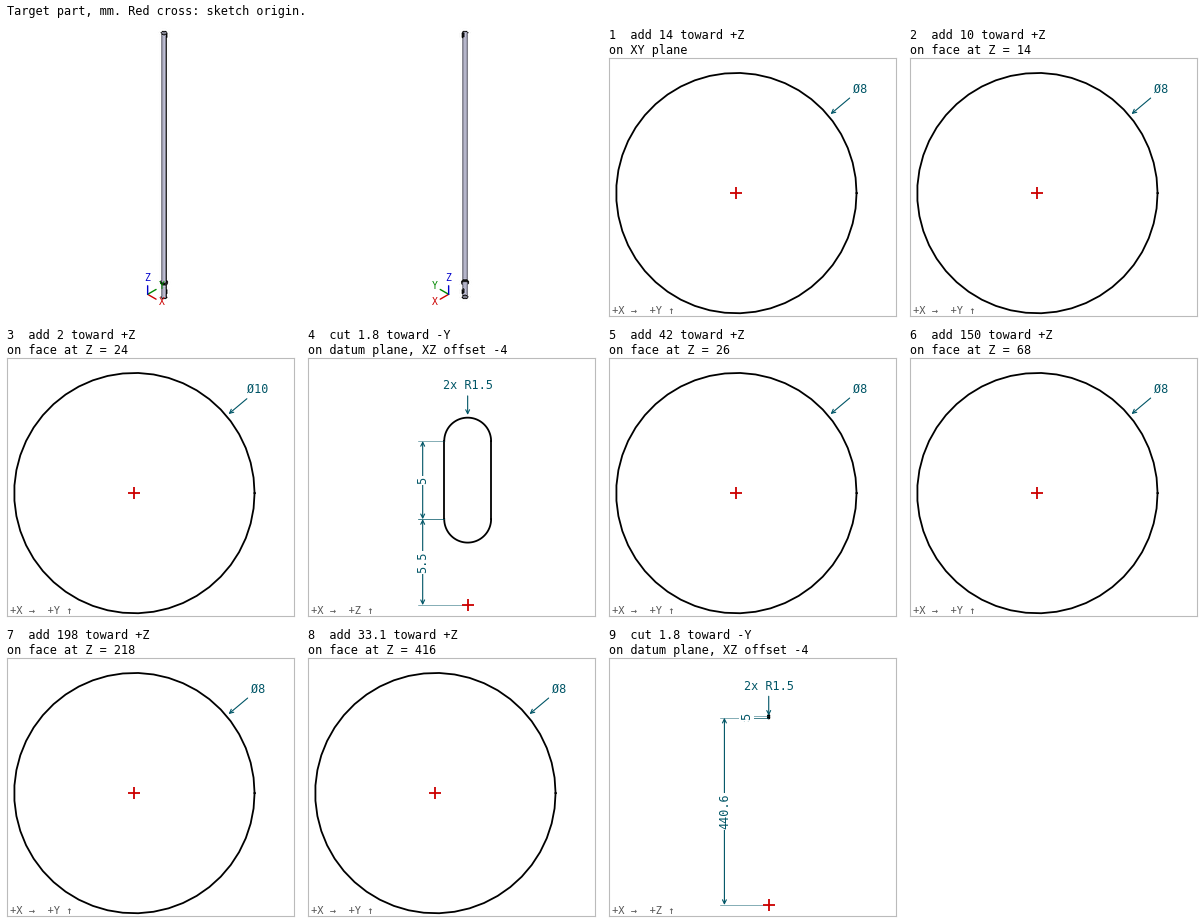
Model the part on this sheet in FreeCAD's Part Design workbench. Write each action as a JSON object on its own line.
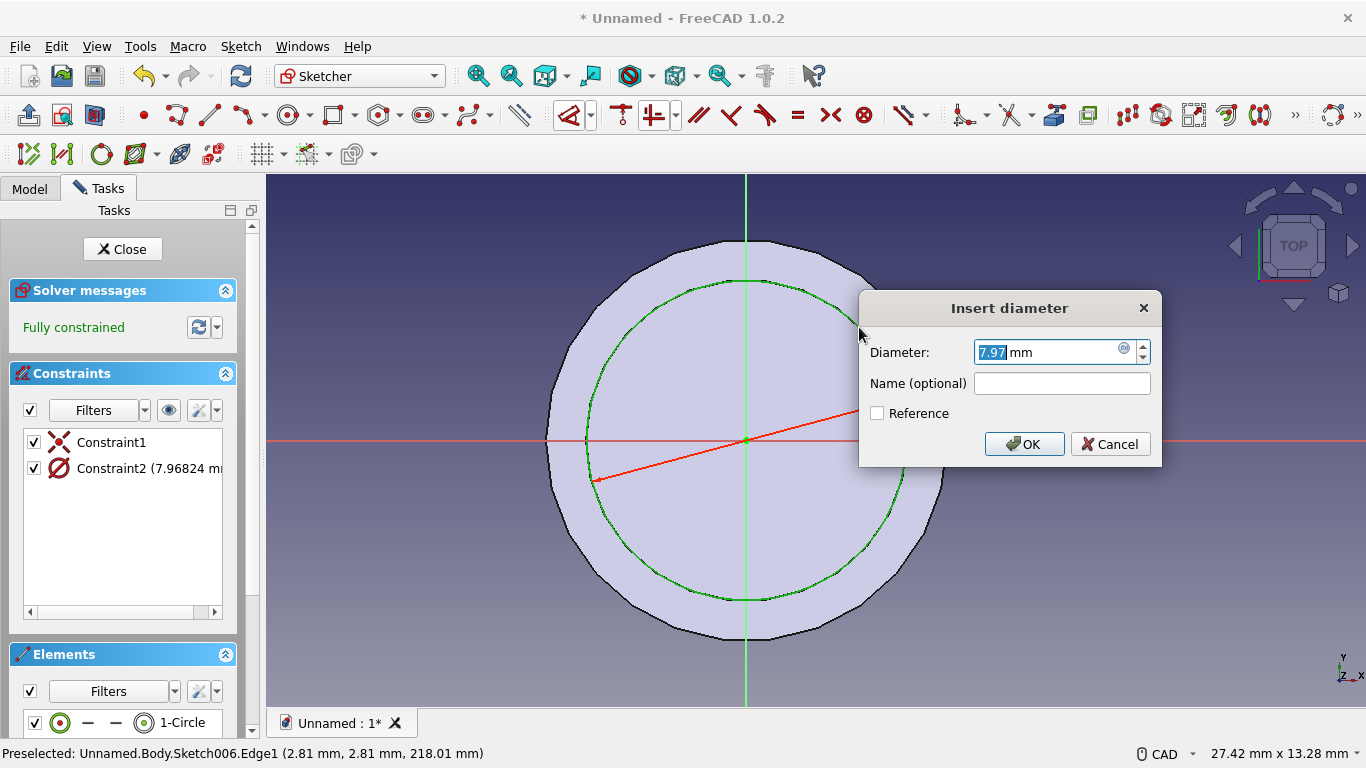
{"action": "type", "text": "8"}
{"action": "key", "text": "Return"}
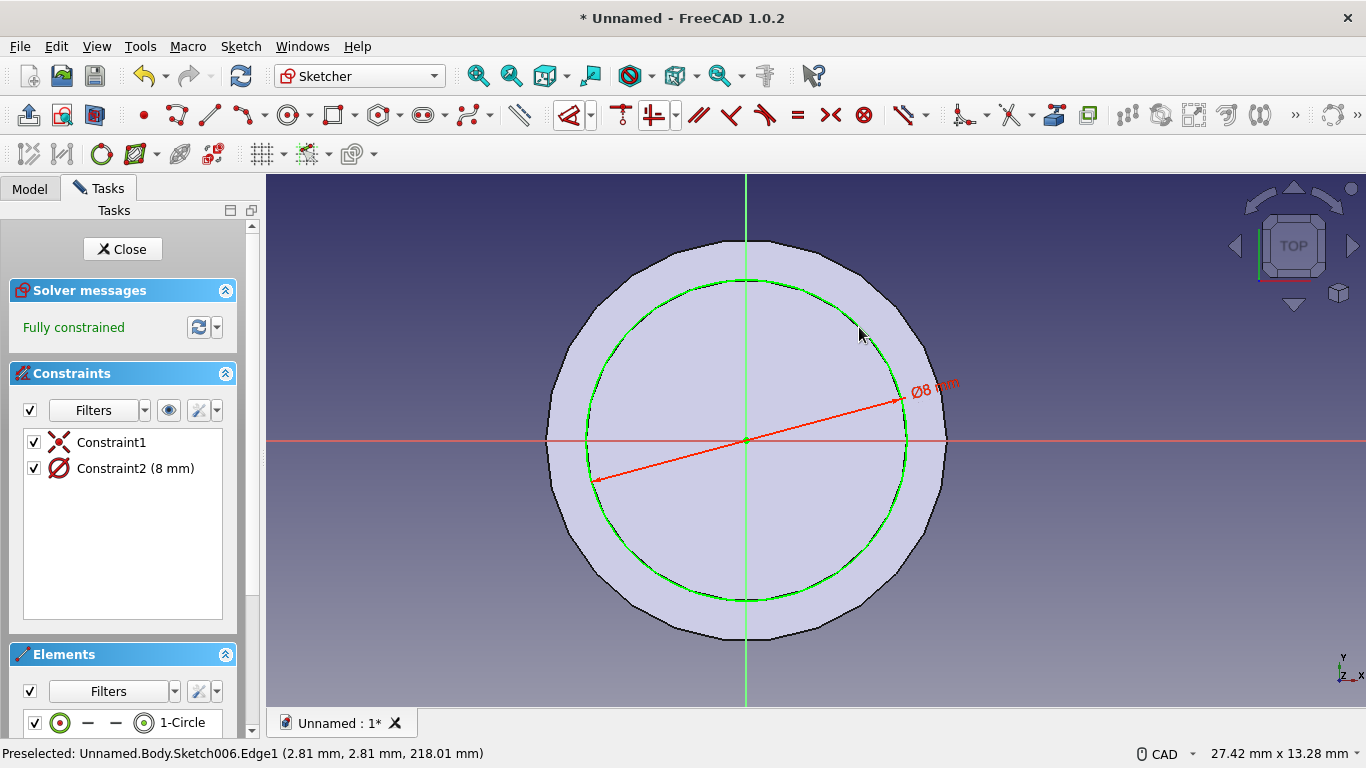
{"action": "left_click", "coordinate": [123, 249]}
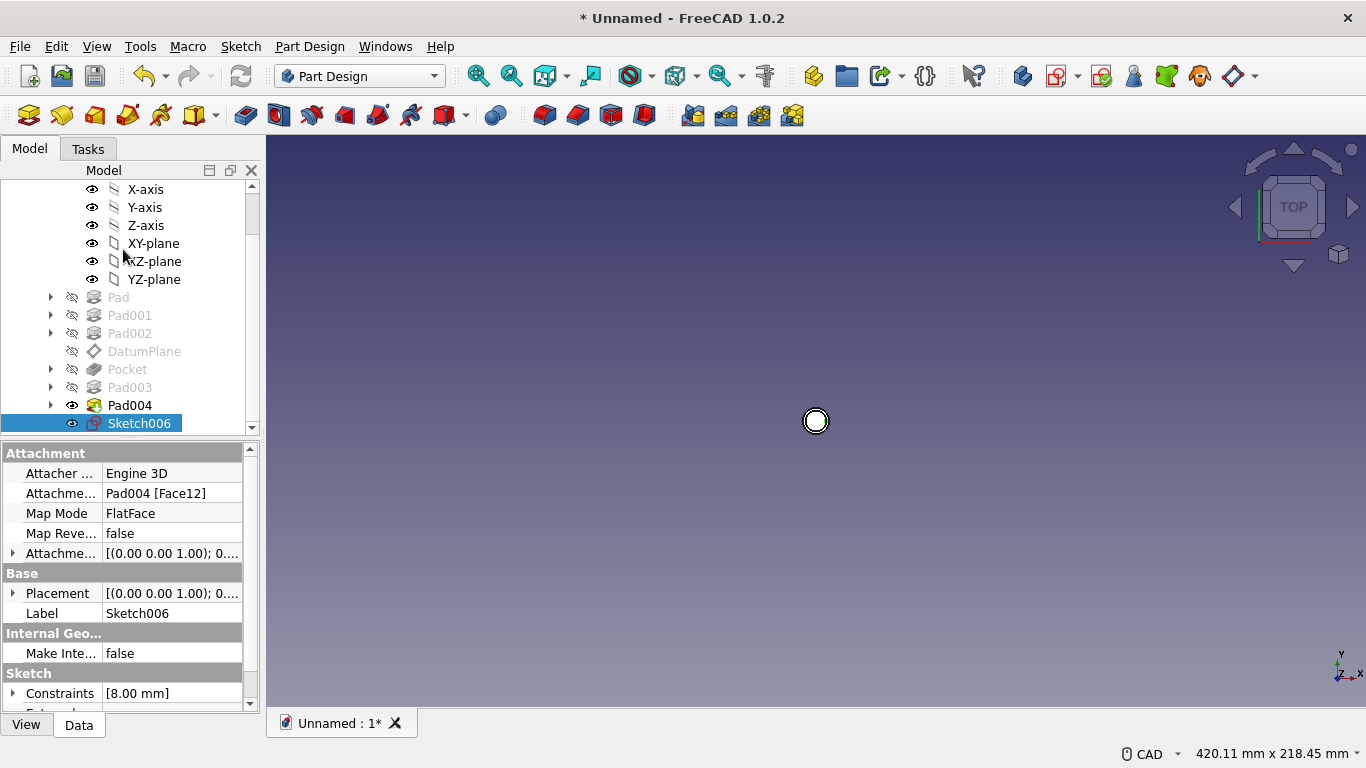
{"action": "left_click", "coordinate": [29, 116]}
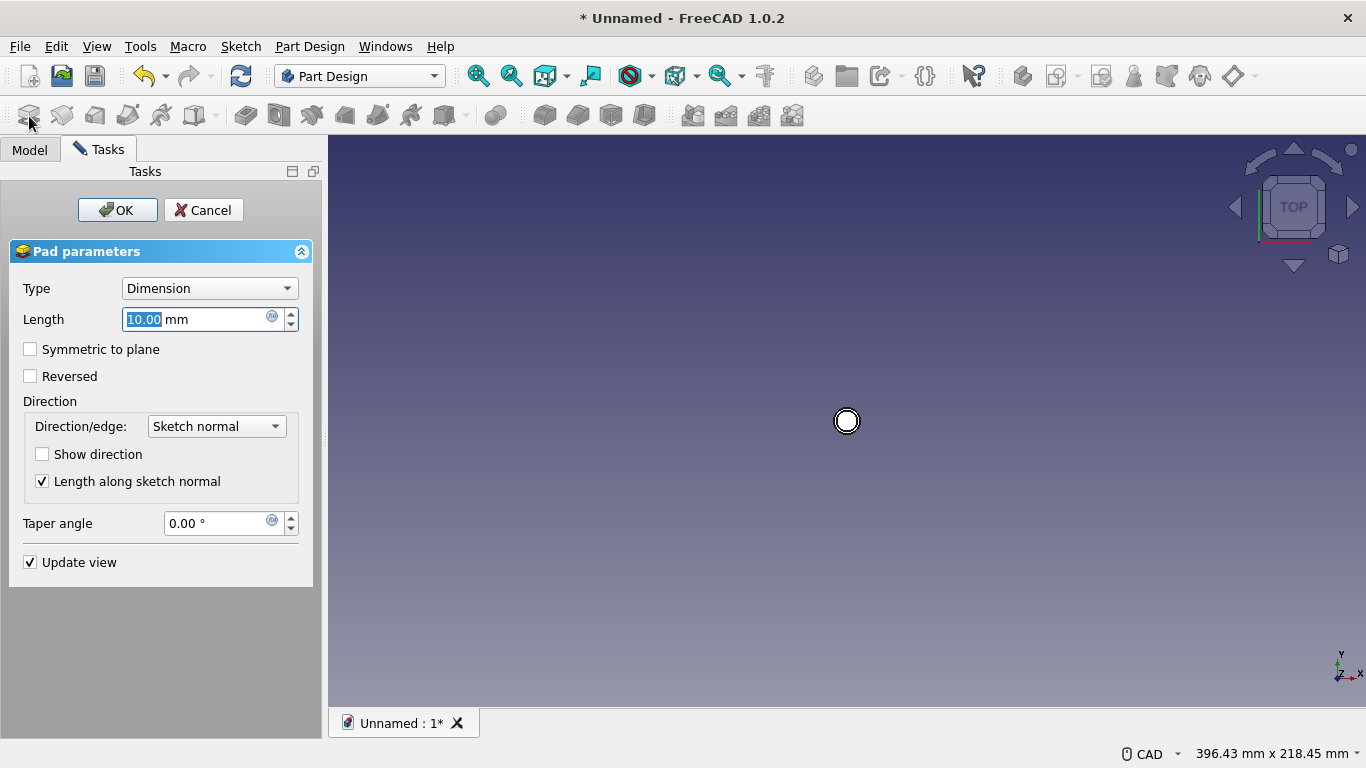
{"action": "type", "text": "198"}
{"action": "key", "text": "Tab"}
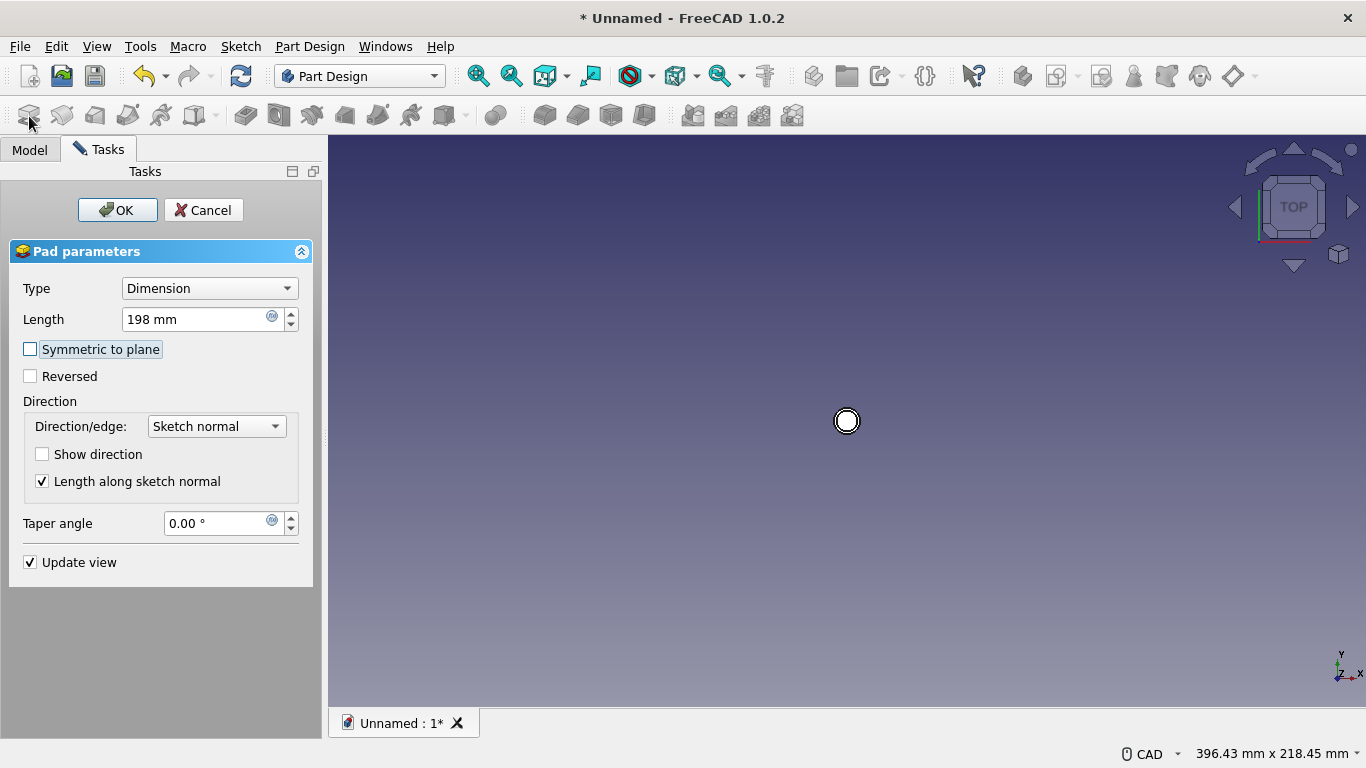
{"action": "left_click", "coordinate": [118, 210]}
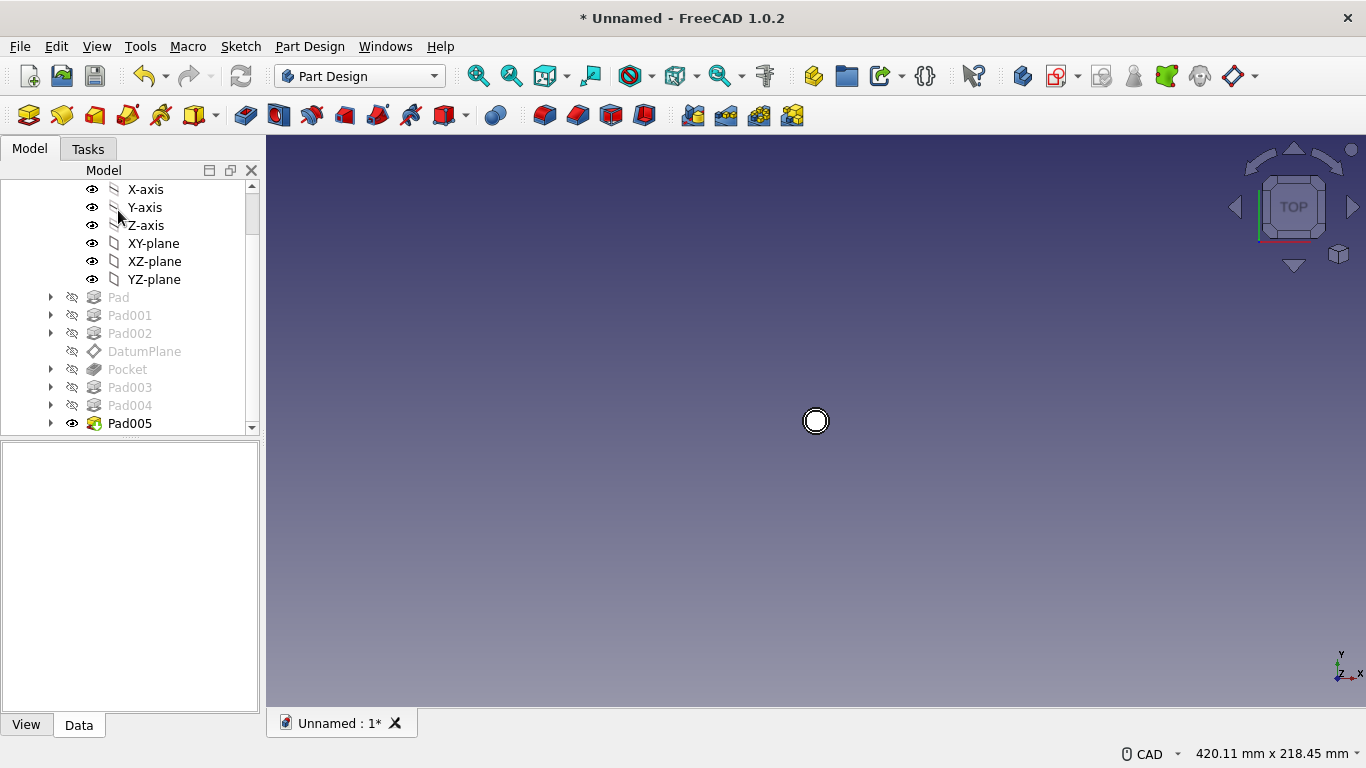
{"action": "left_click", "coordinate": [479, 76]}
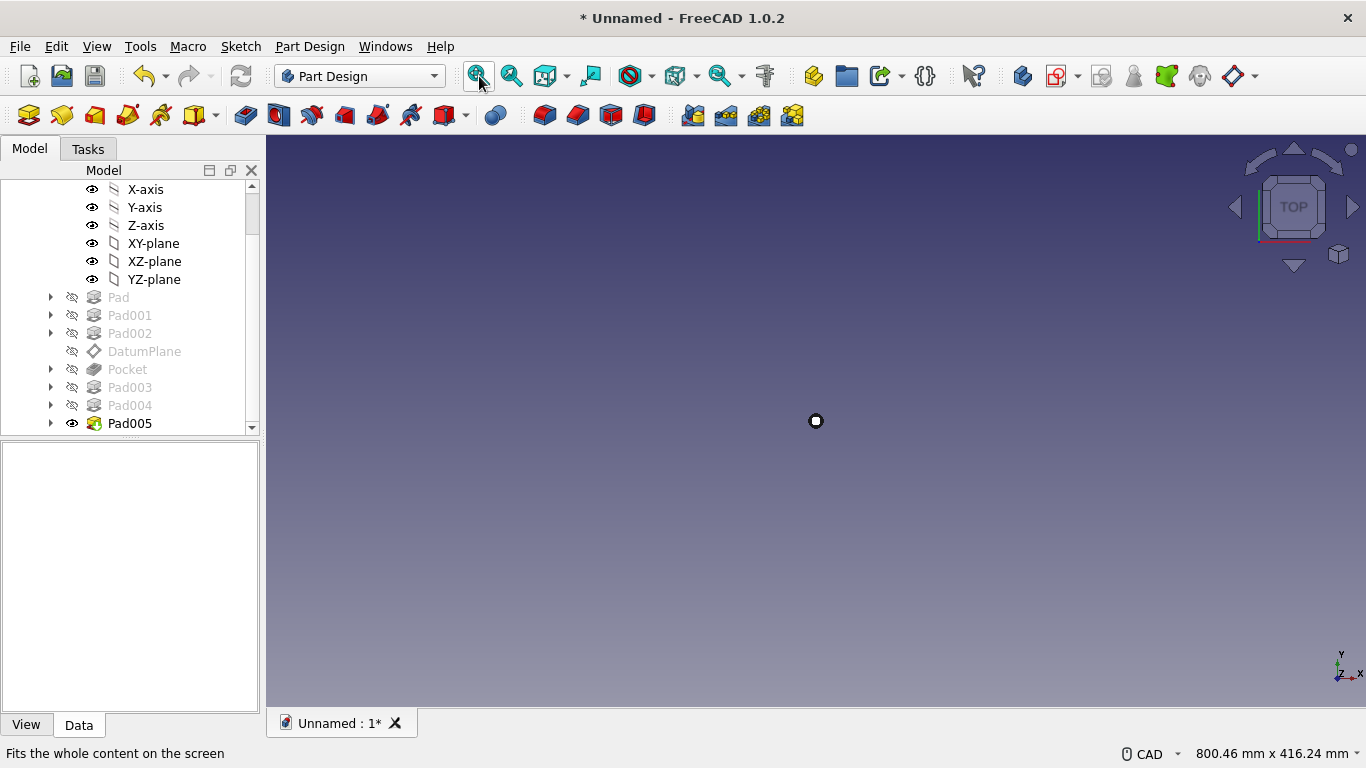
{"action": "scroll", "coordinate": [816, 420], "scroll_direction": "up", "scroll_amount": 4}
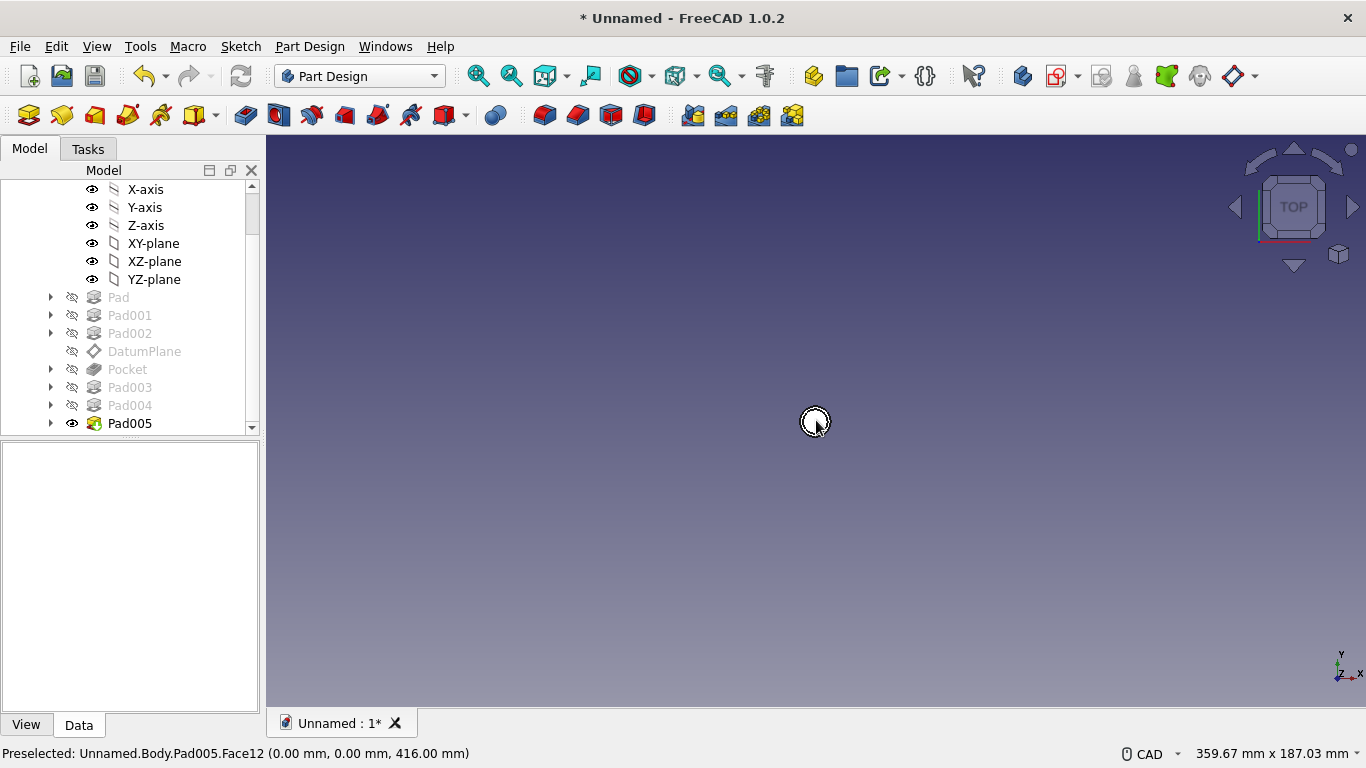
{"action": "left_click", "coordinate": [815, 421]}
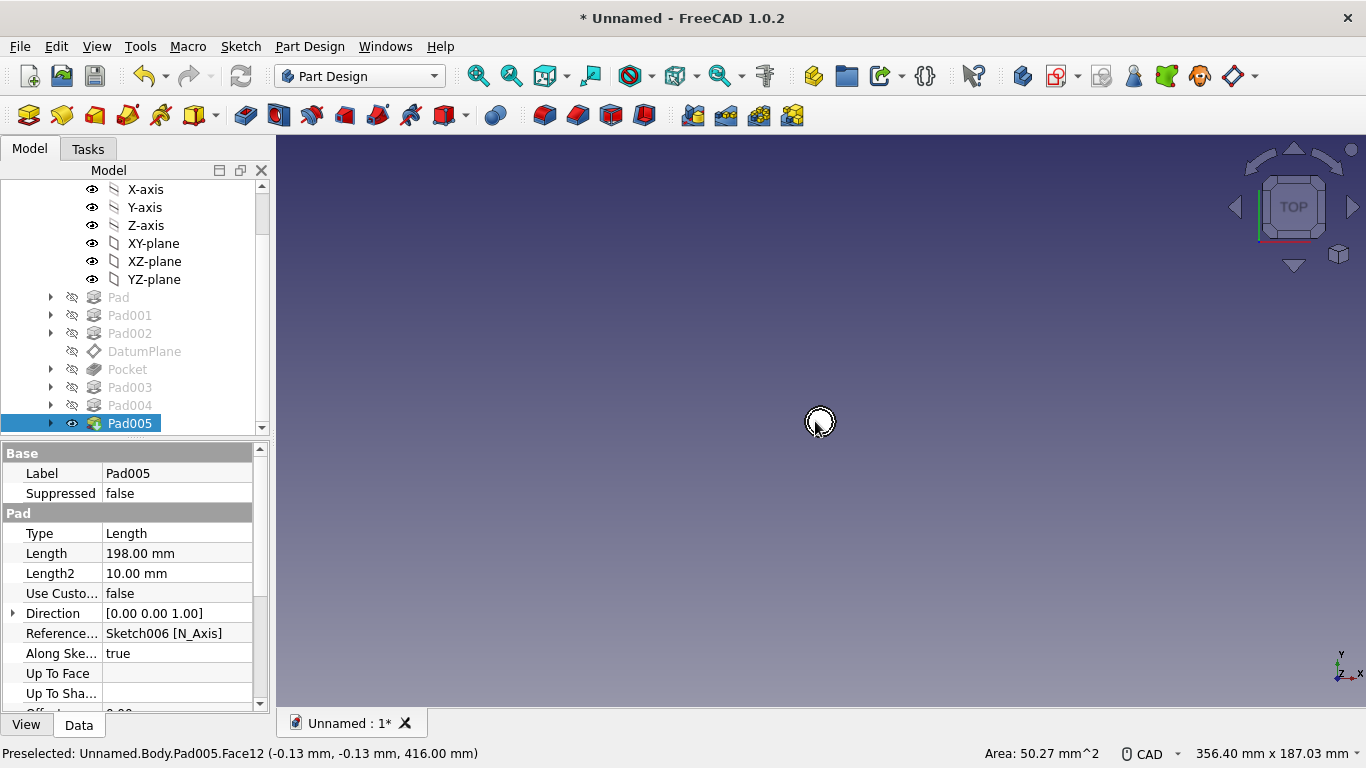
{"action": "left_click", "coordinate": [1056, 76]}